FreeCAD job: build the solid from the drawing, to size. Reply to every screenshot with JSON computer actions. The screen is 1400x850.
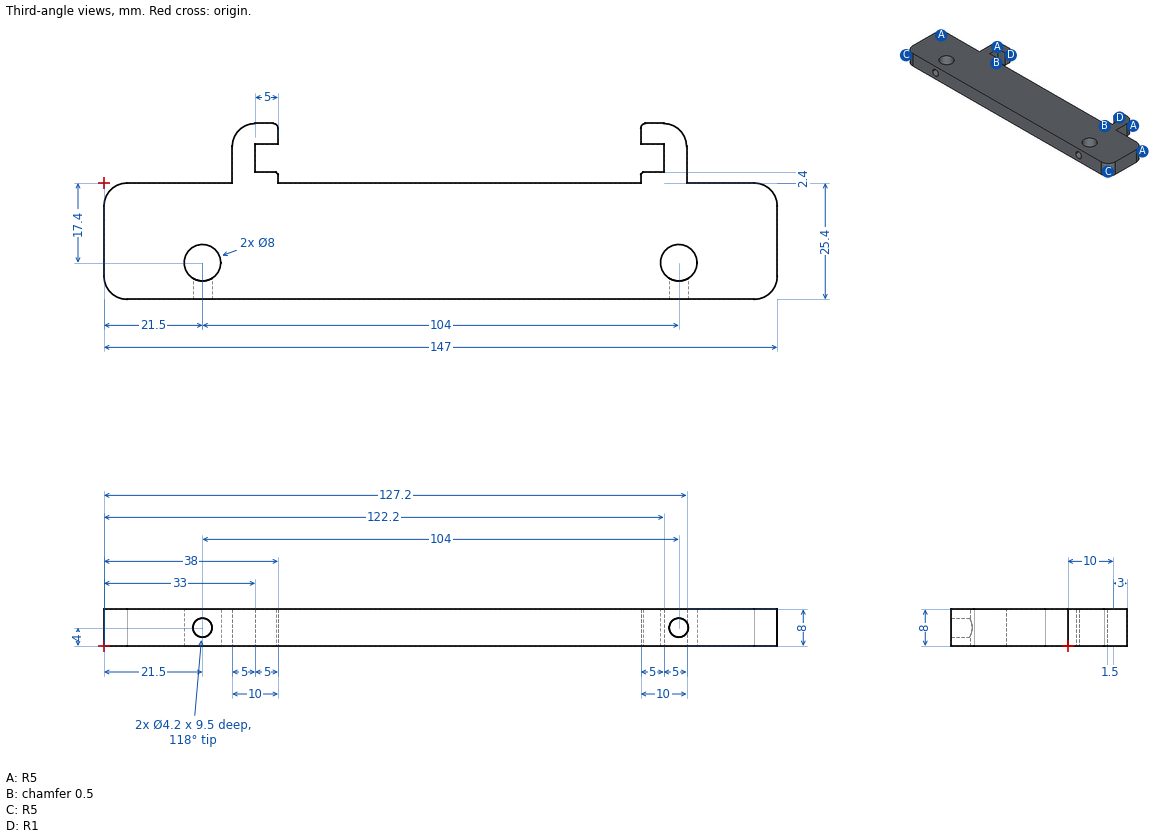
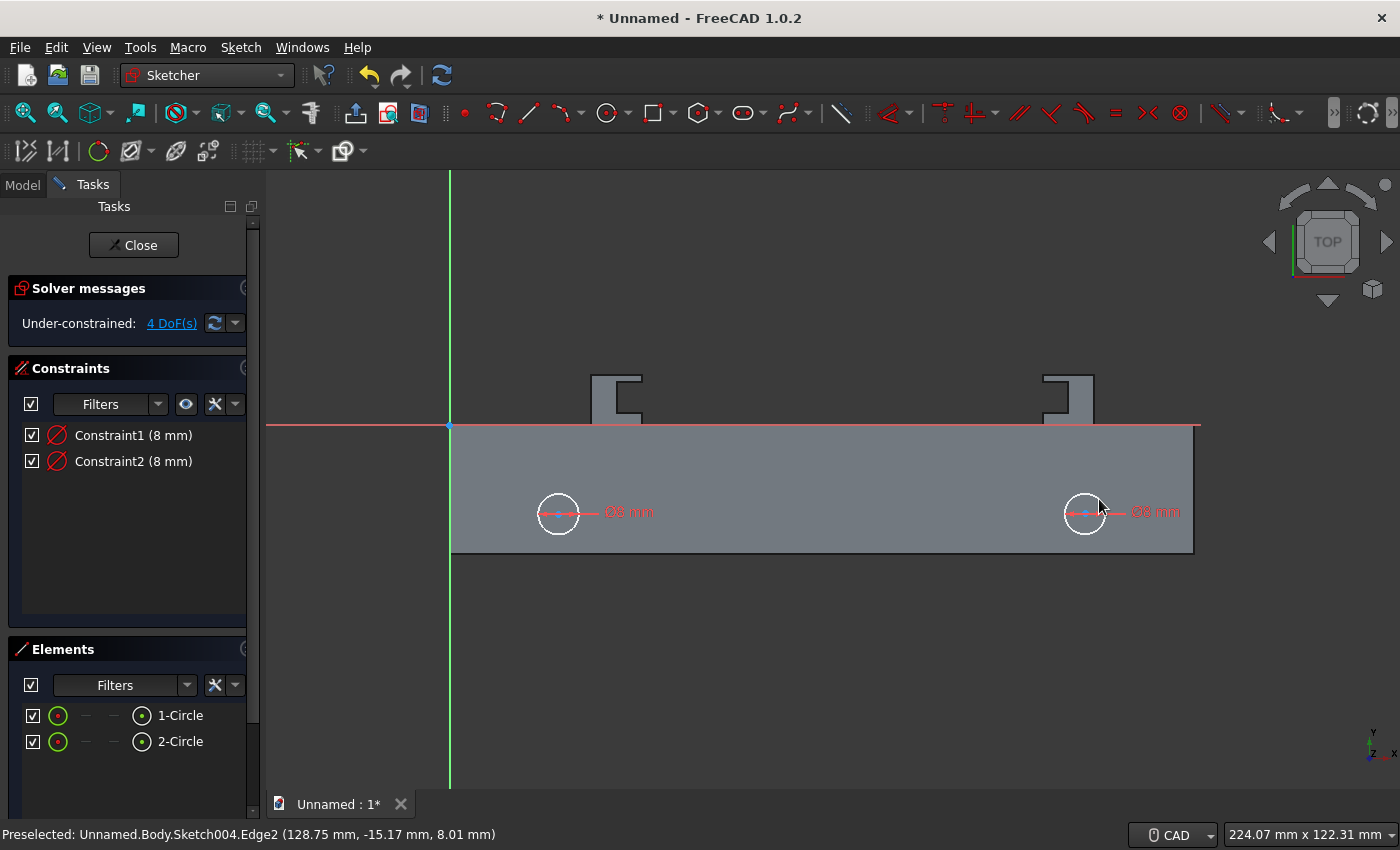
{"action": "left_click", "coordinate": [888, 114]}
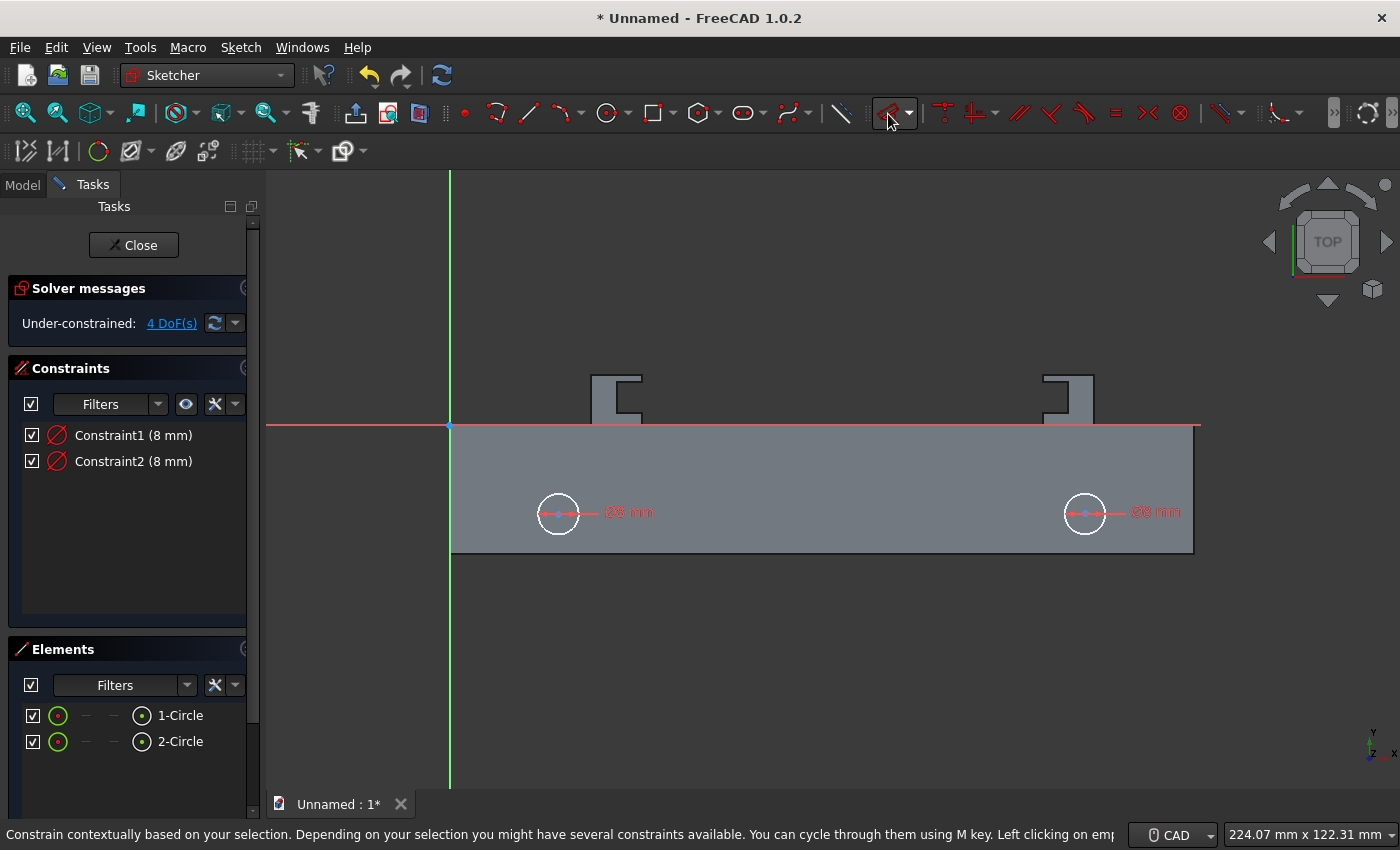
{"action": "left_click", "coordinate": [558, 514]}
{"action": "left_click", "coordinate": [504, 391]}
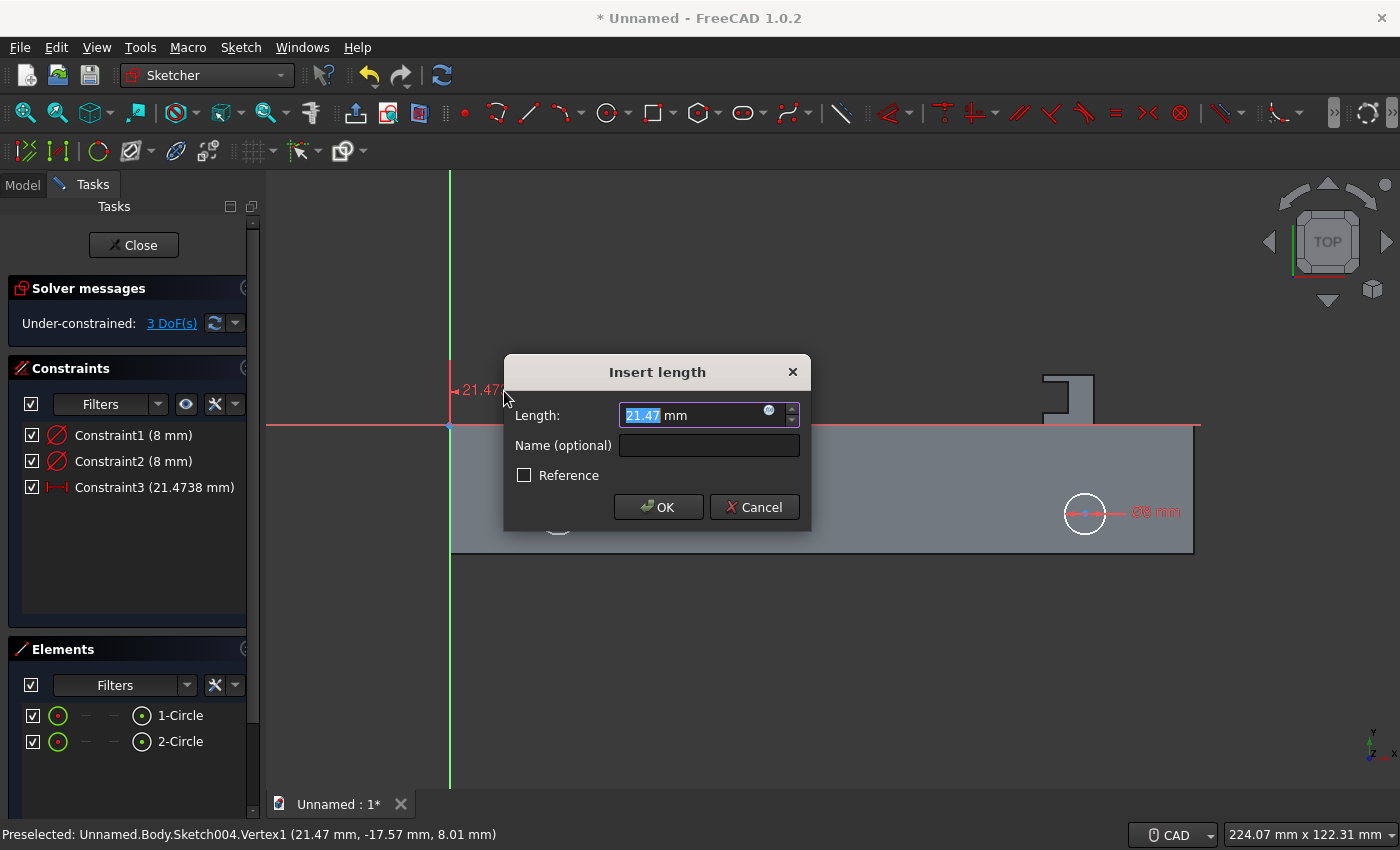
{"action": "type", "text": "21.5"}
{"action": "key", "text": "Return"}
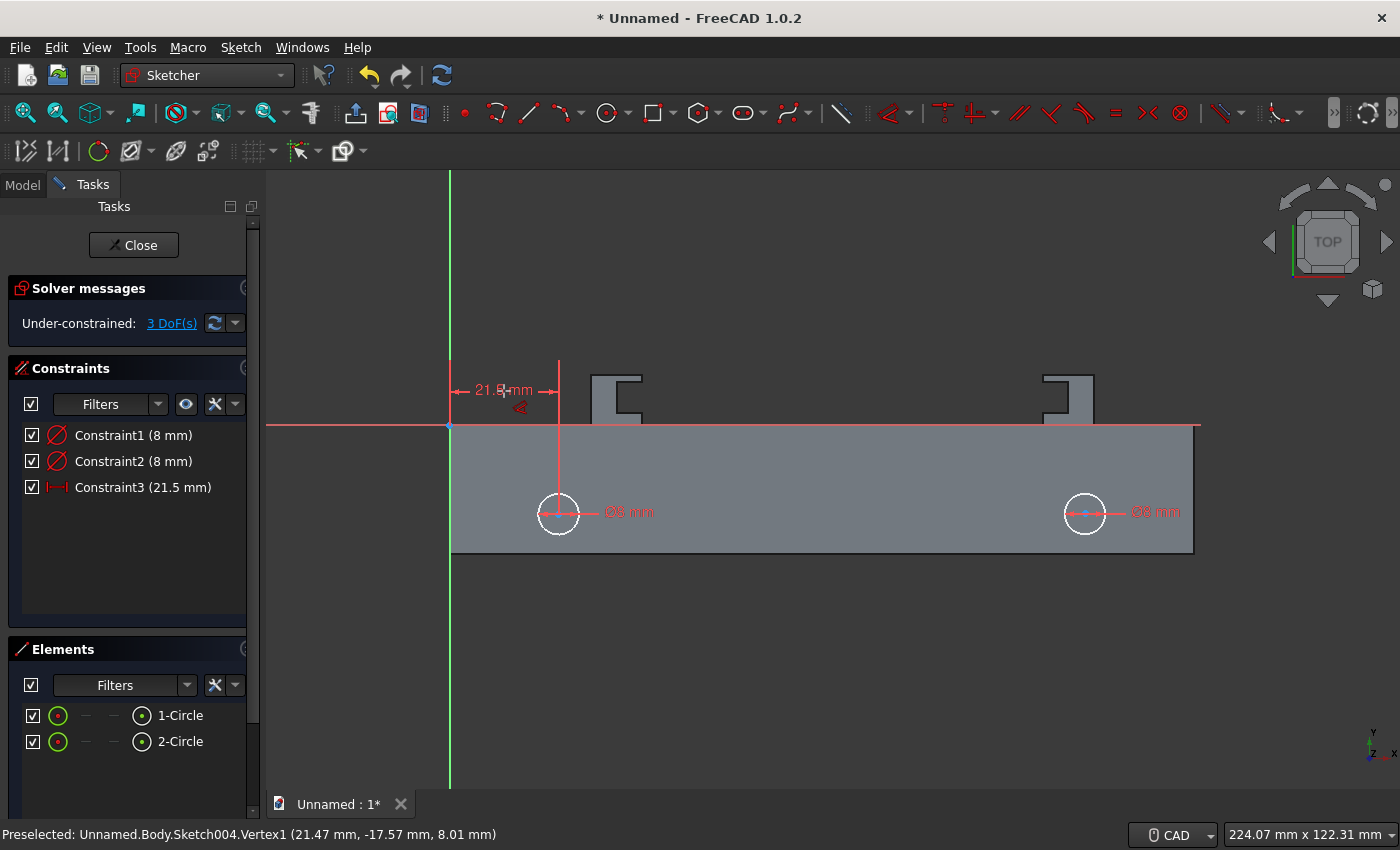
{"action": "left_click", "coordinate": [559, 514]}
{"action": "left_click", "coordinate": [416, 470]}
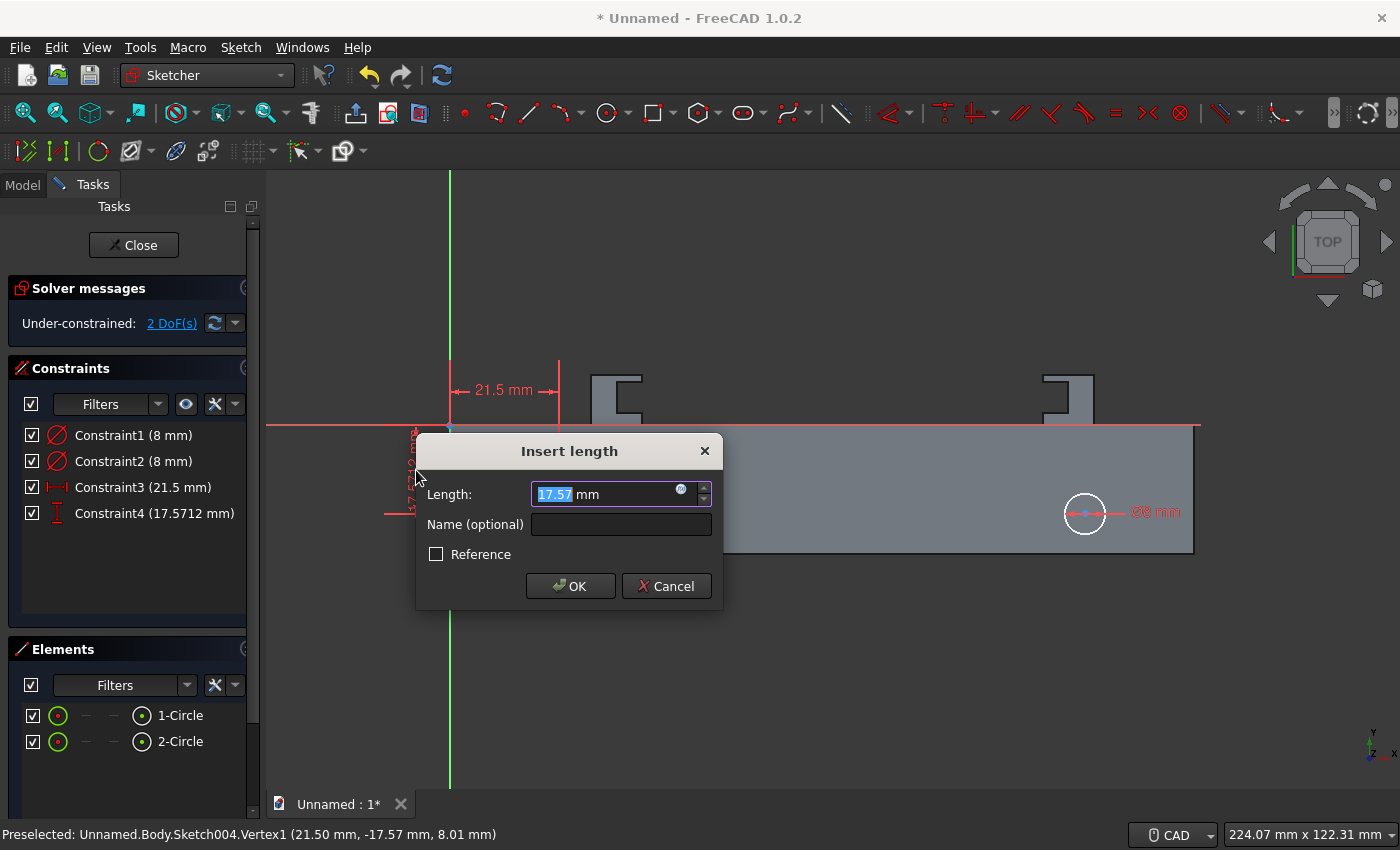
{"action": "type", "text": "17.4"}
{"action": "key", "text": "Return"}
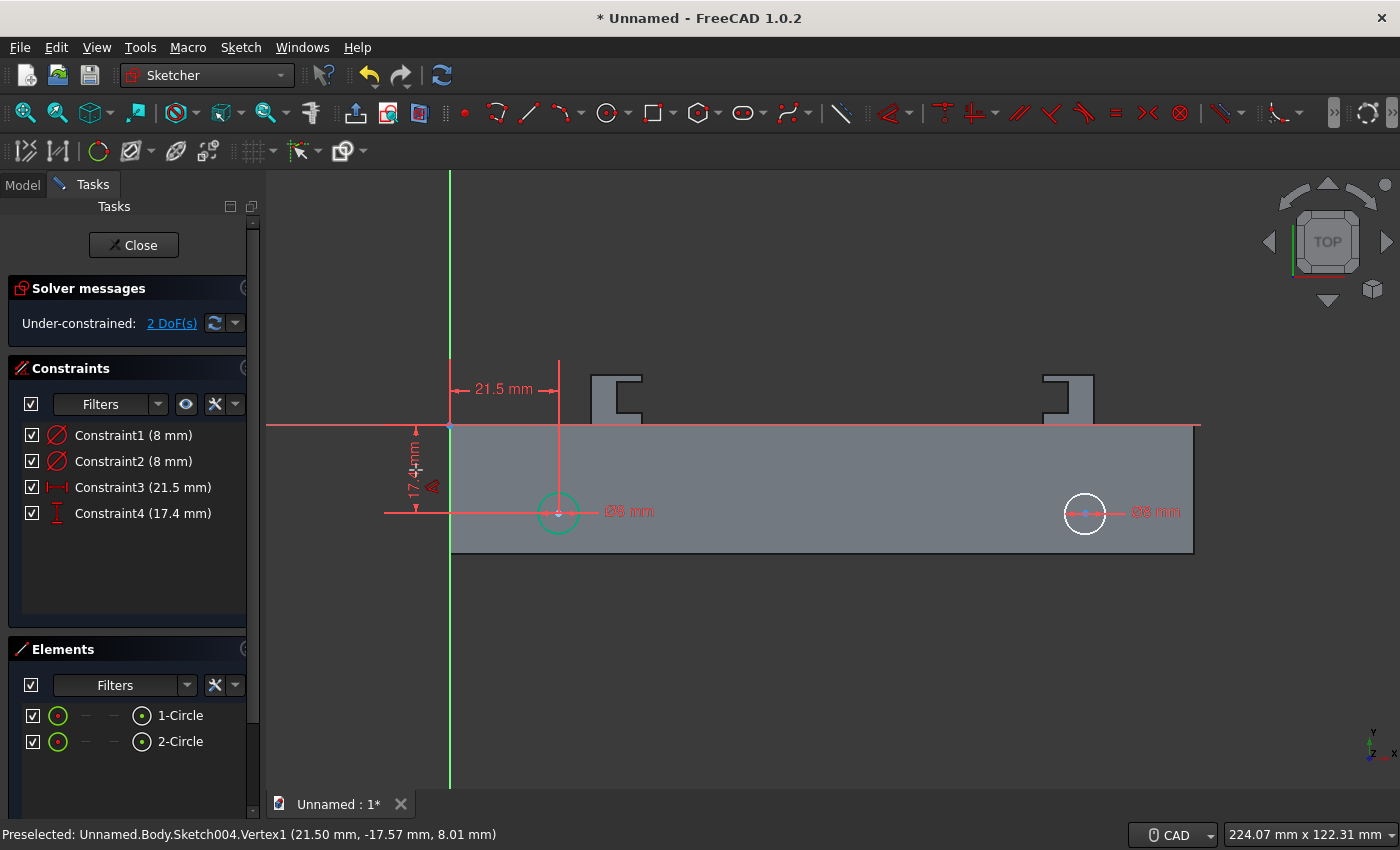
{"action": "left_click", "coordinate": [1085, 514]}
{"action": "left_click", "coordinate": [416, 449]}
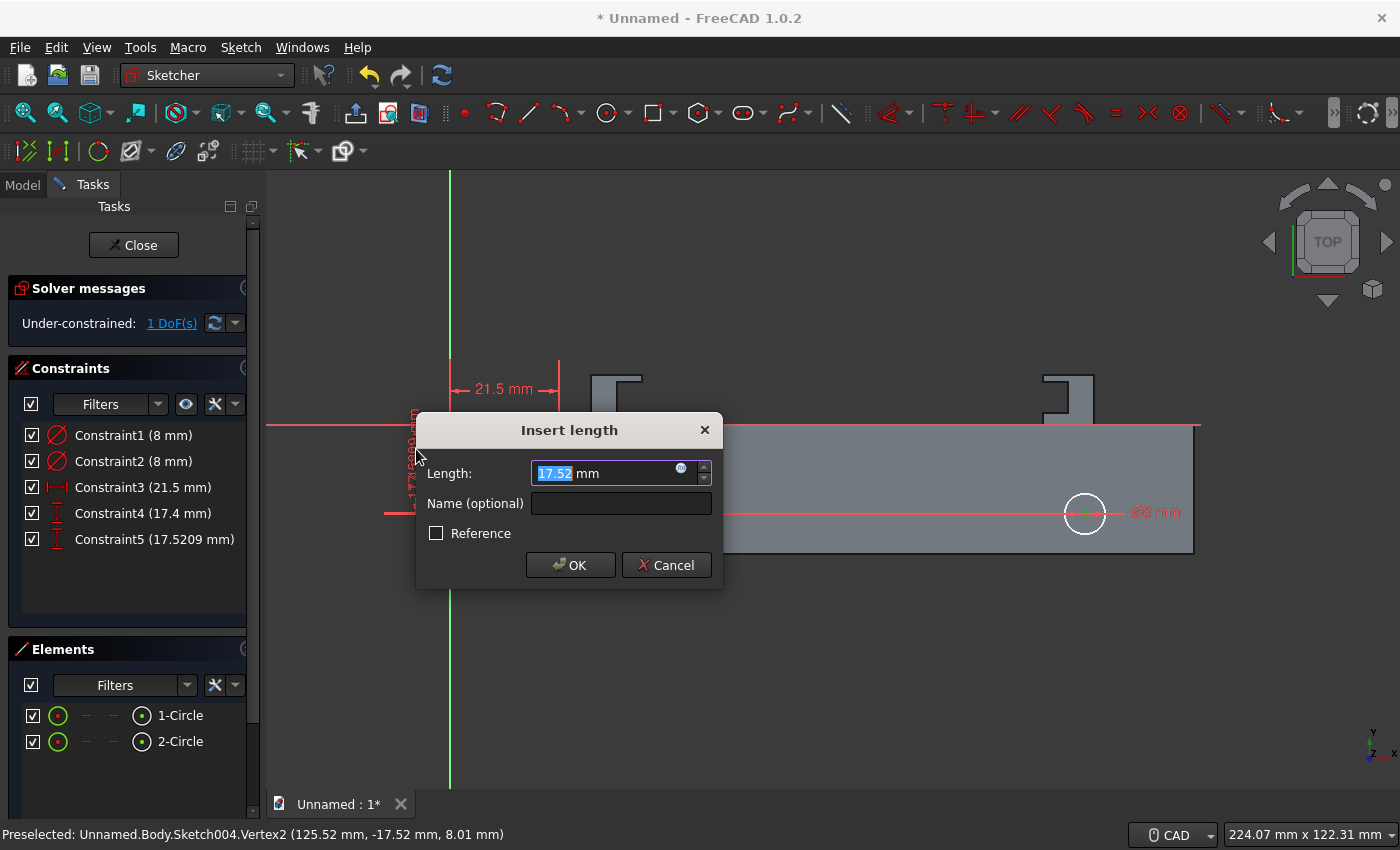
{"action": "type", "text": "17.4"}
{"action": "key", "text": "Return"}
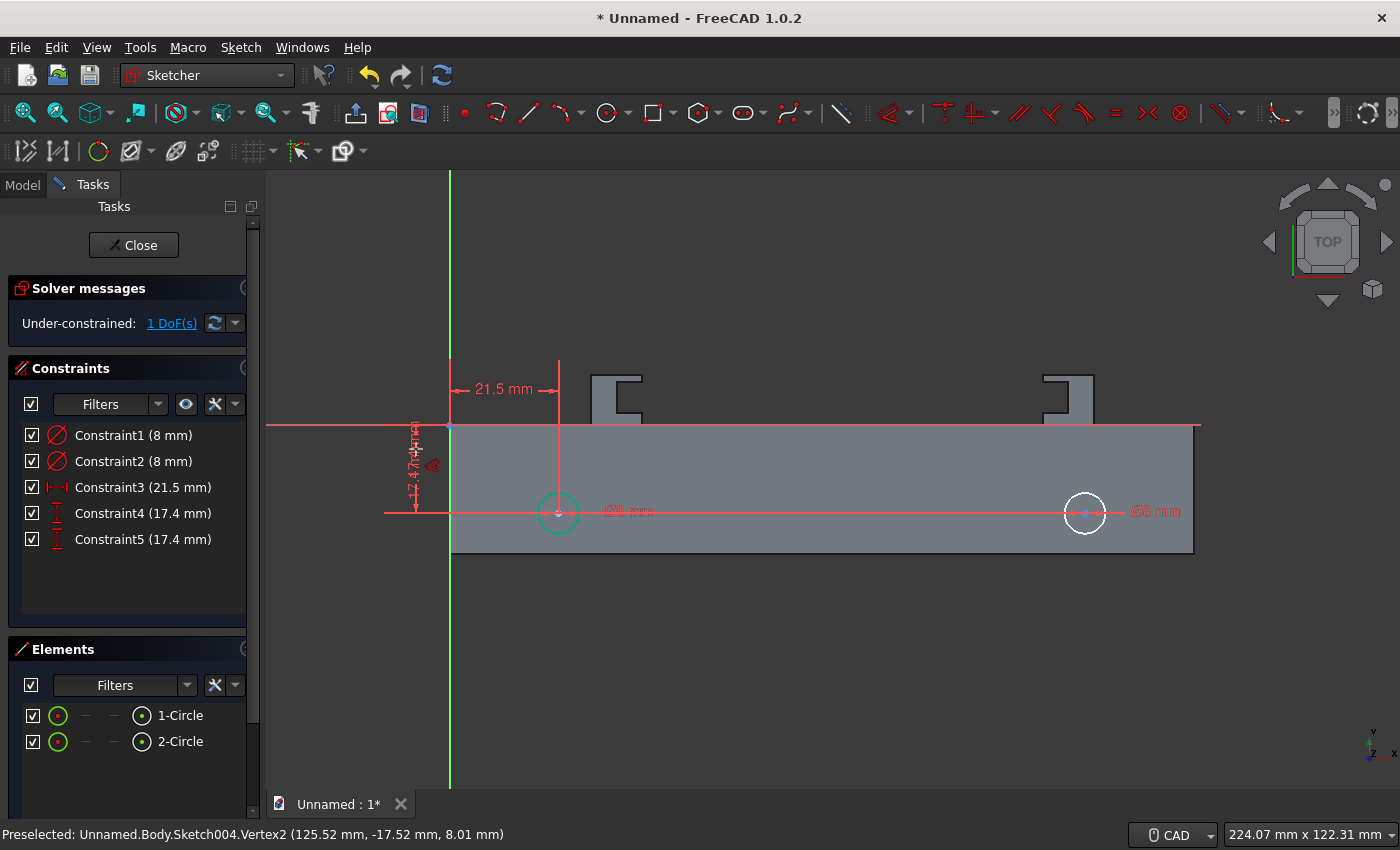
{"action": "left_click", "coordinate": [559, 513]}